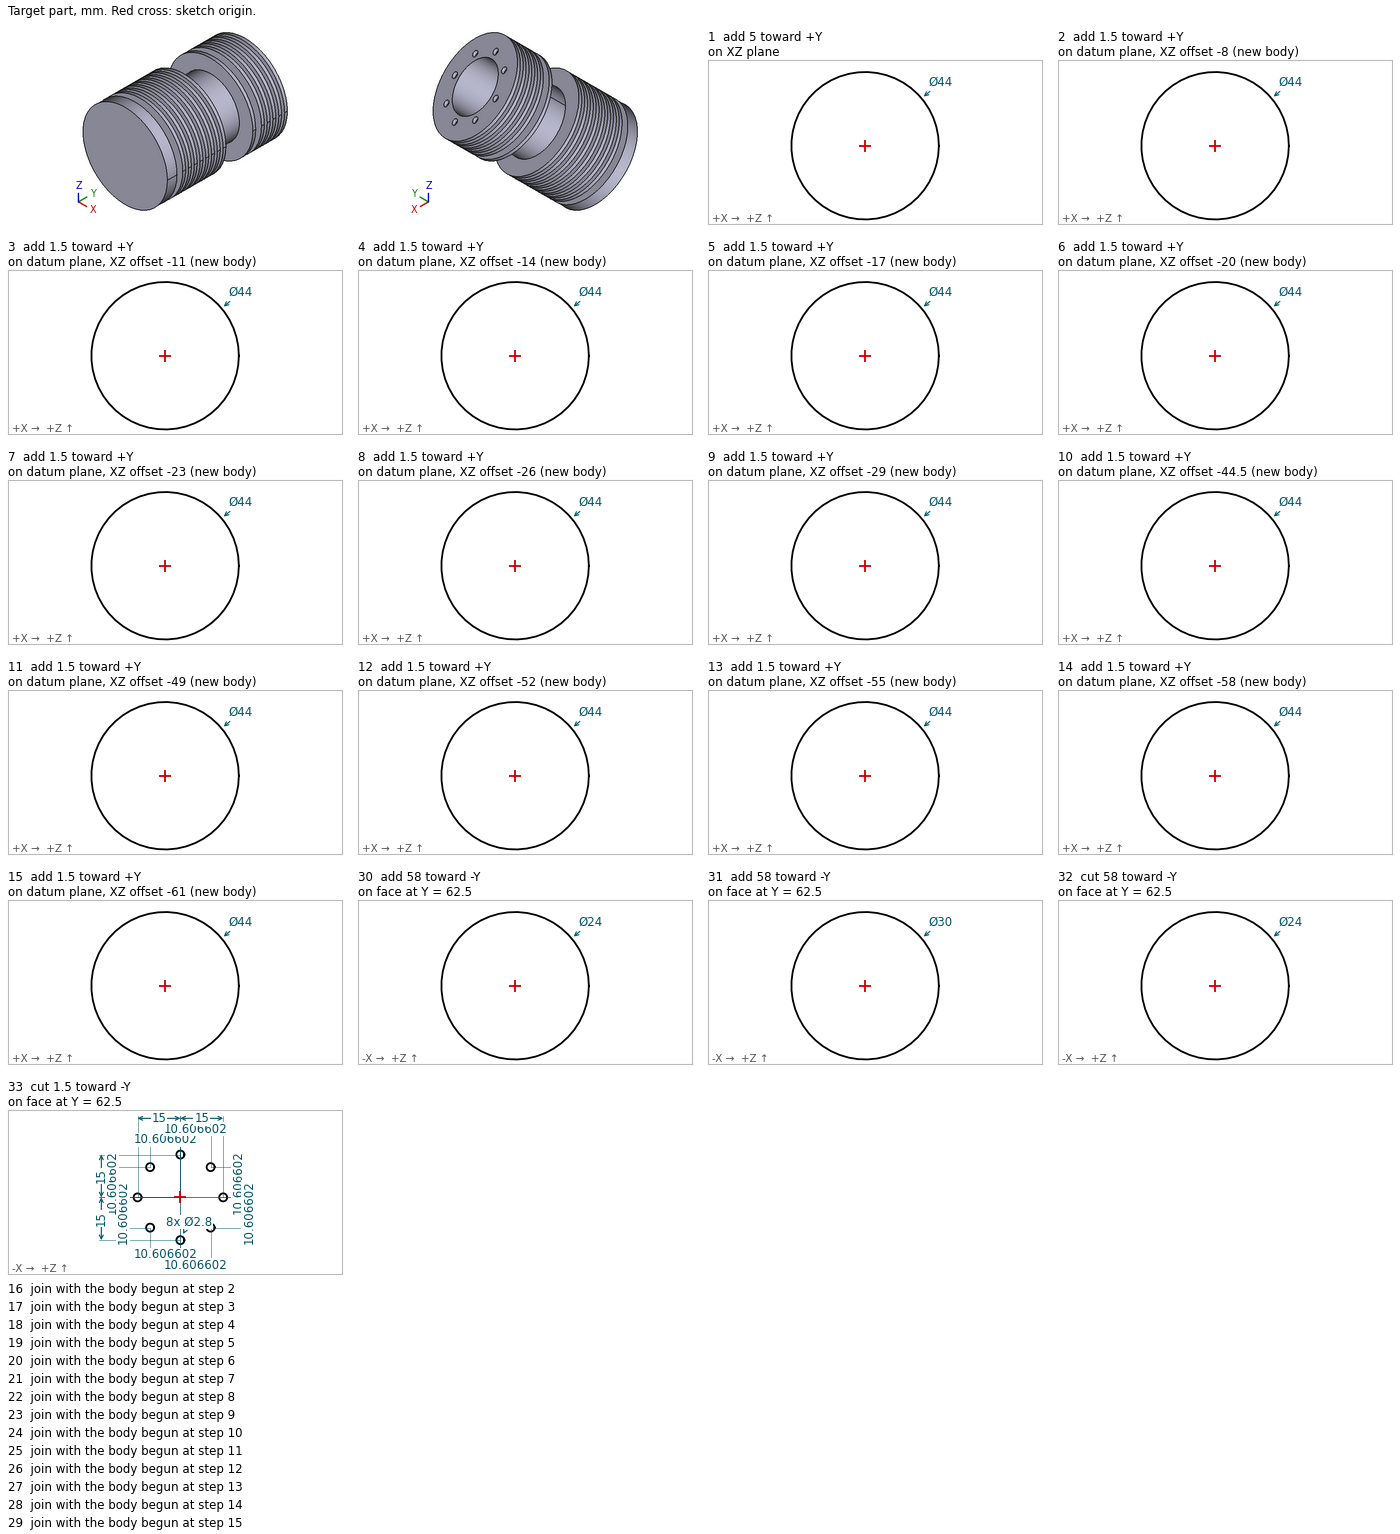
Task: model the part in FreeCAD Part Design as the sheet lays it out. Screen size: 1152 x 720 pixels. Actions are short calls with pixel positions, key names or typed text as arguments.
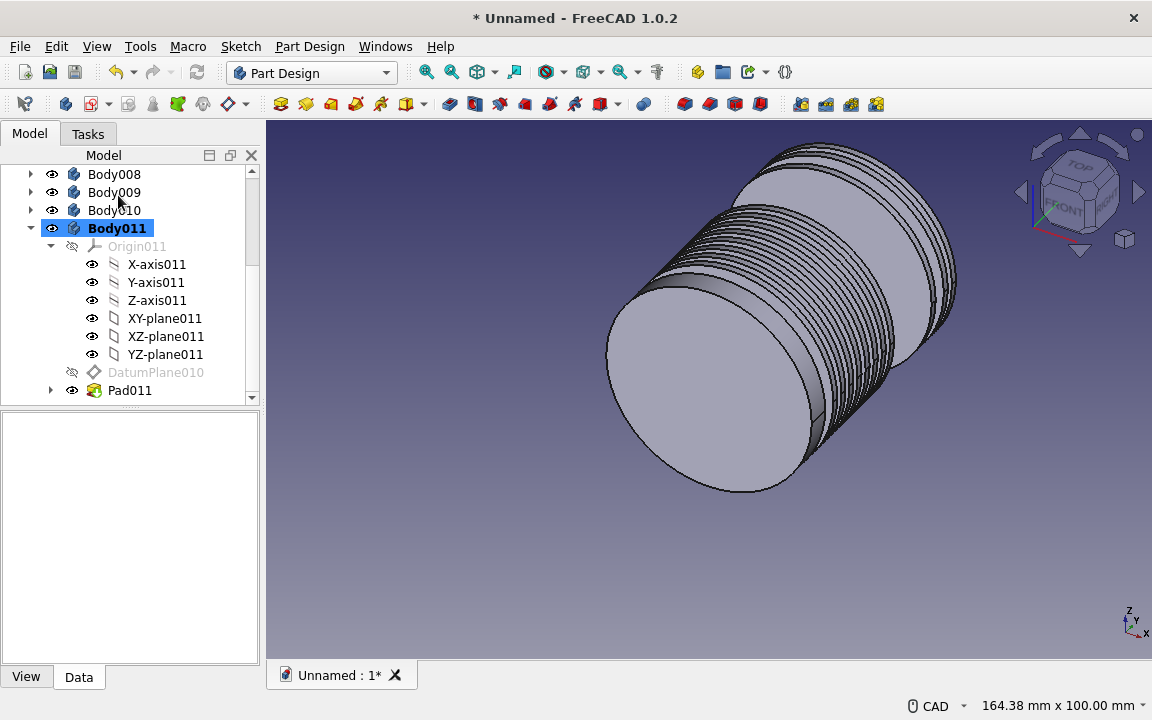
key(v)
key(f)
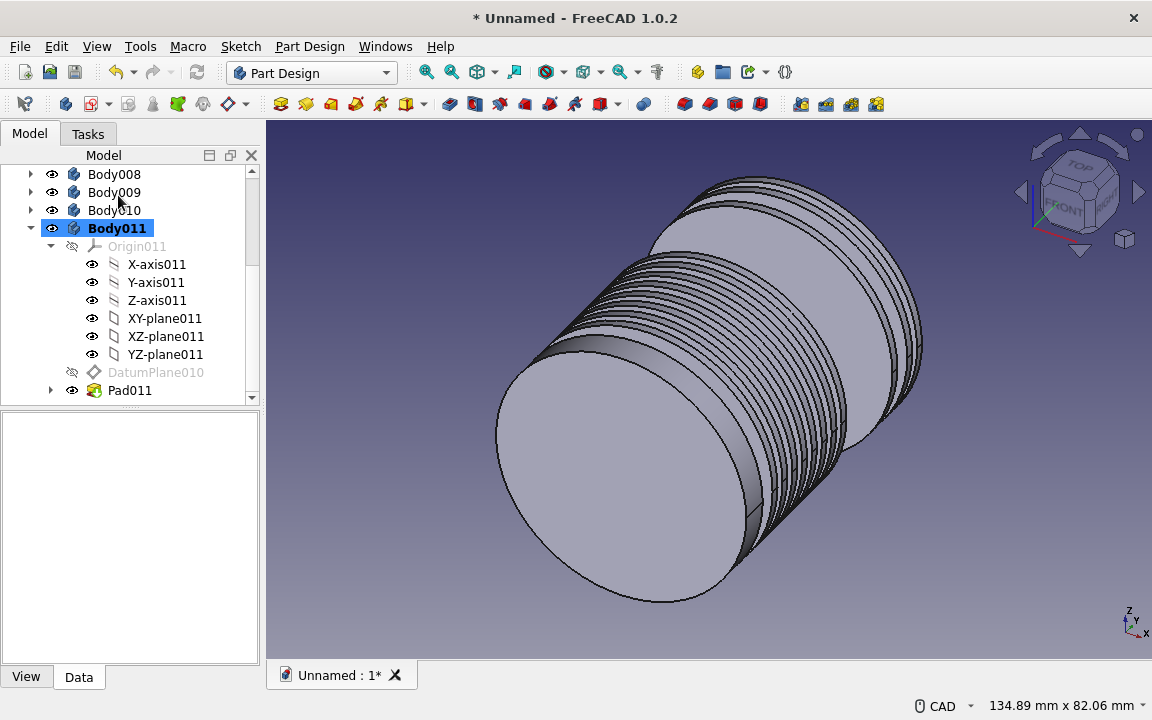
click(66, 104)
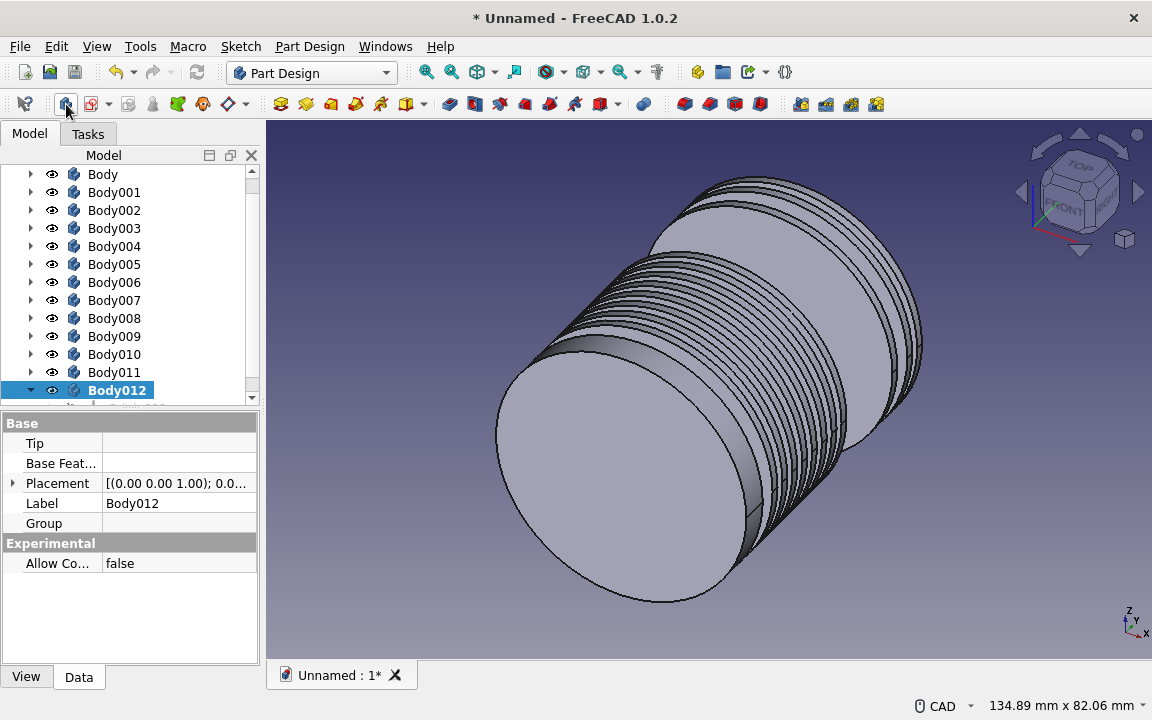
scroll(121, 278, down, 3)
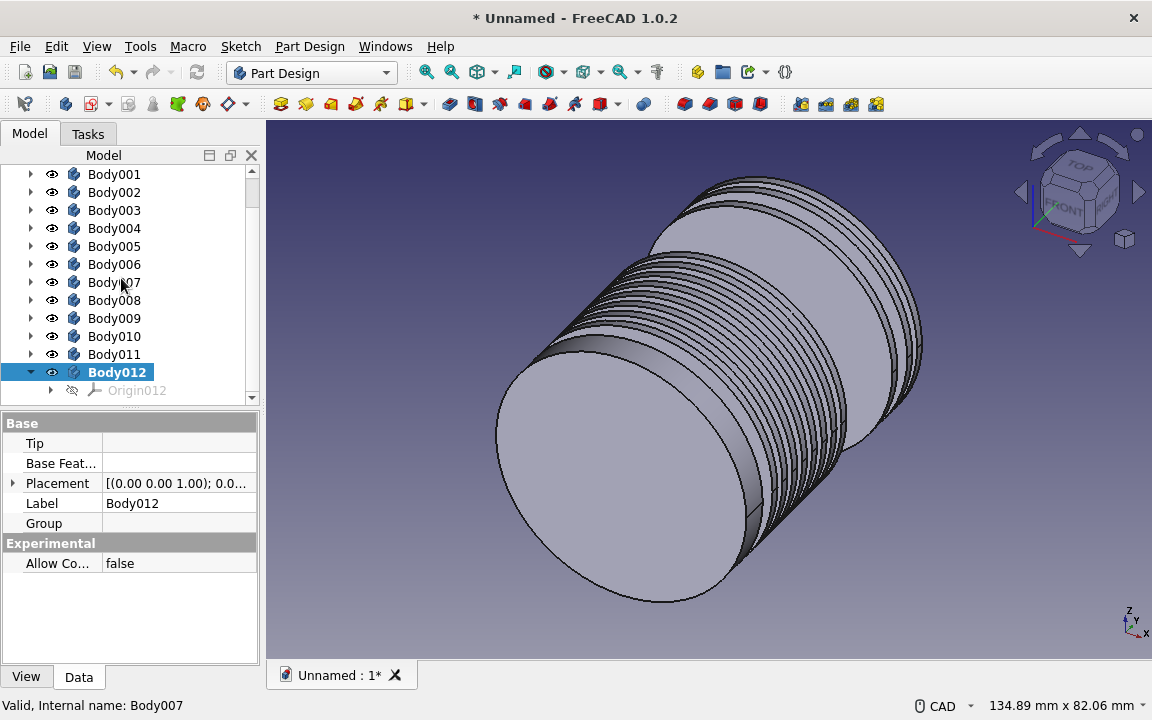
click(51, 390)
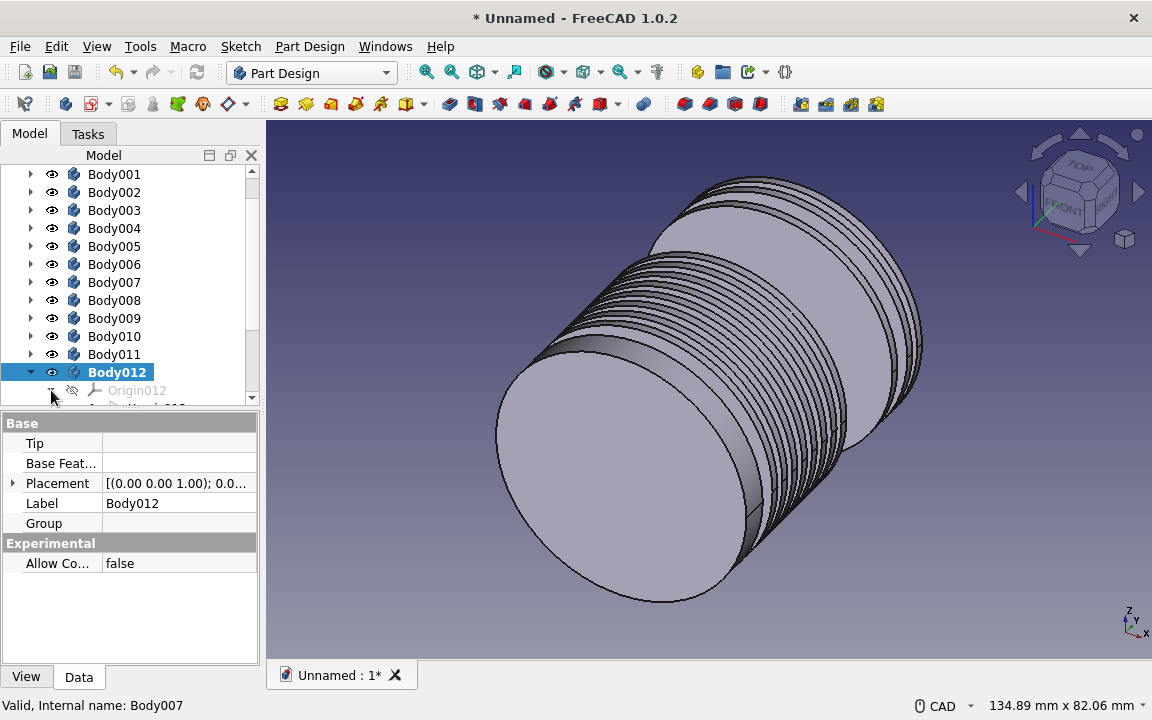
scroll(121, 278, down, 3)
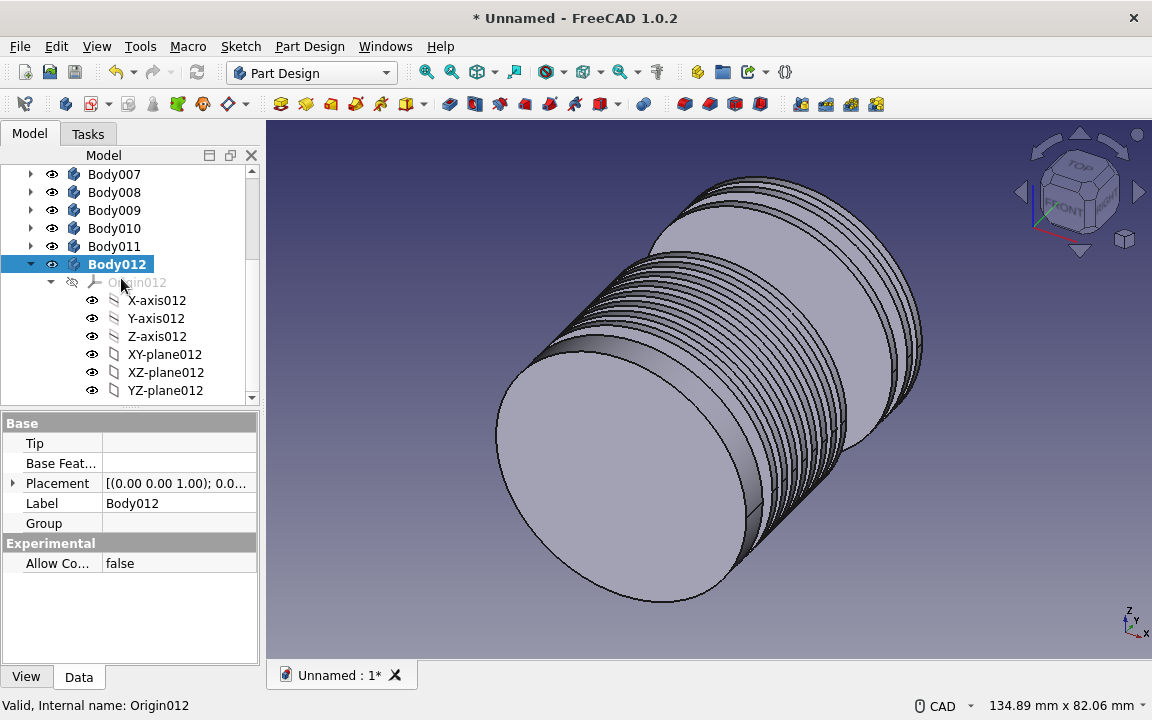
click(137, 372)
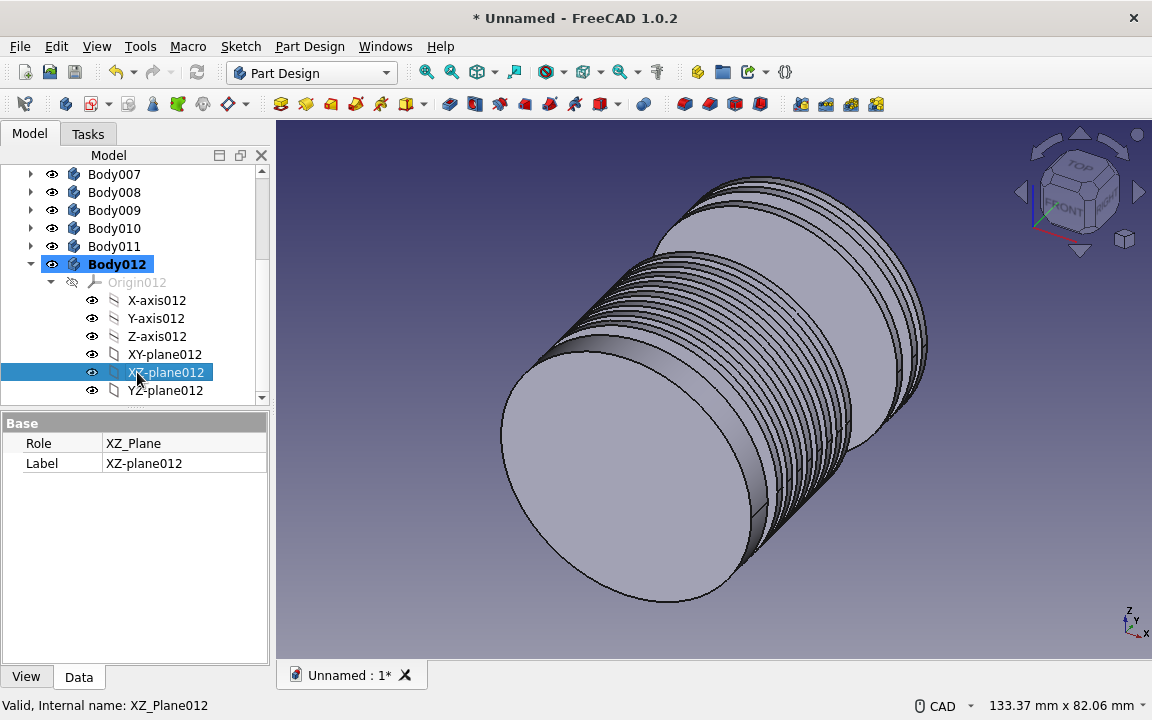
click(228, 104)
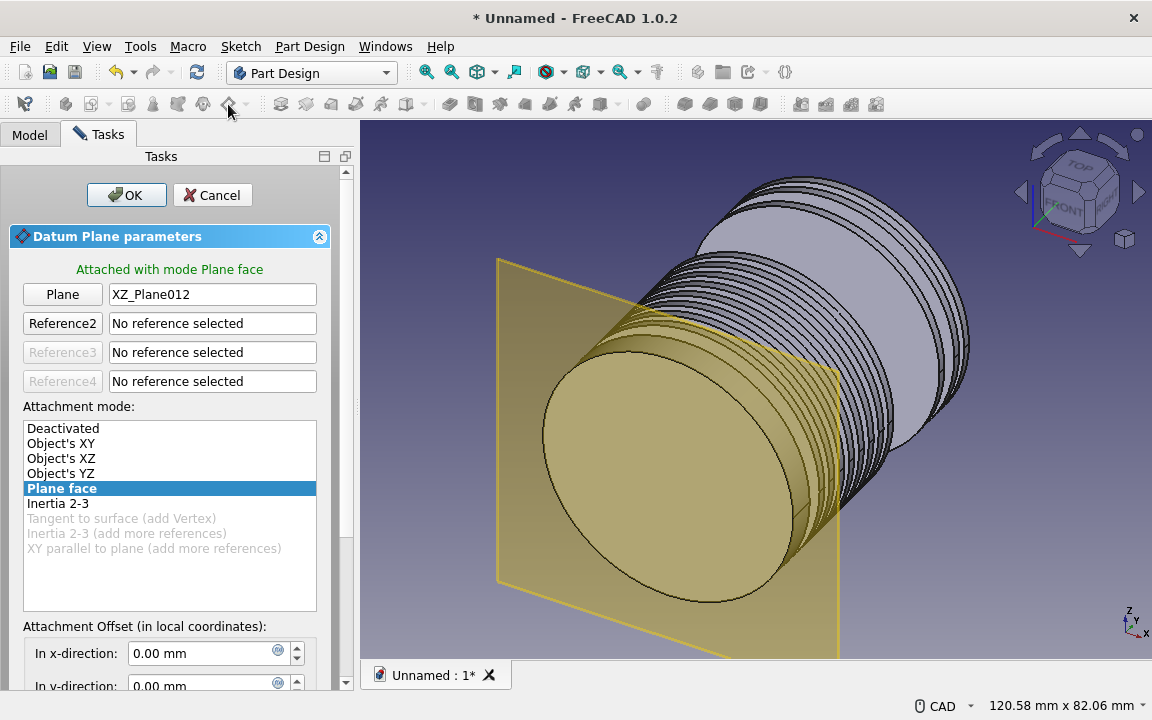
scroll(346, 428, down, 2)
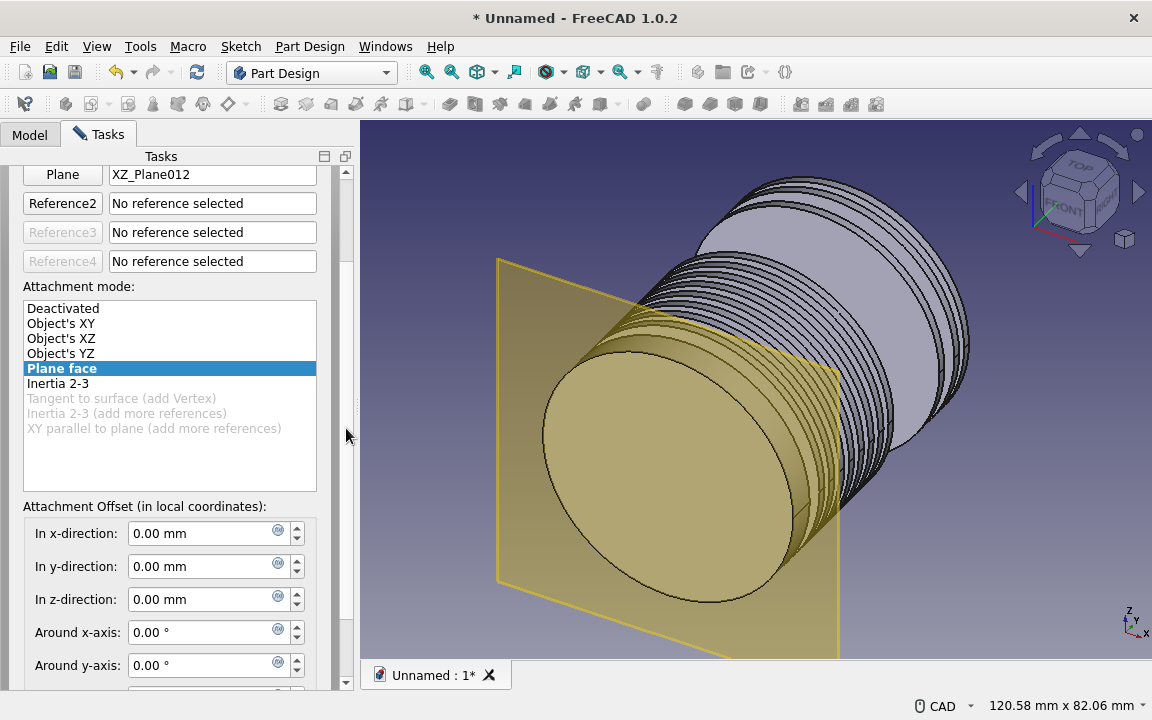
triple_click(210, 600)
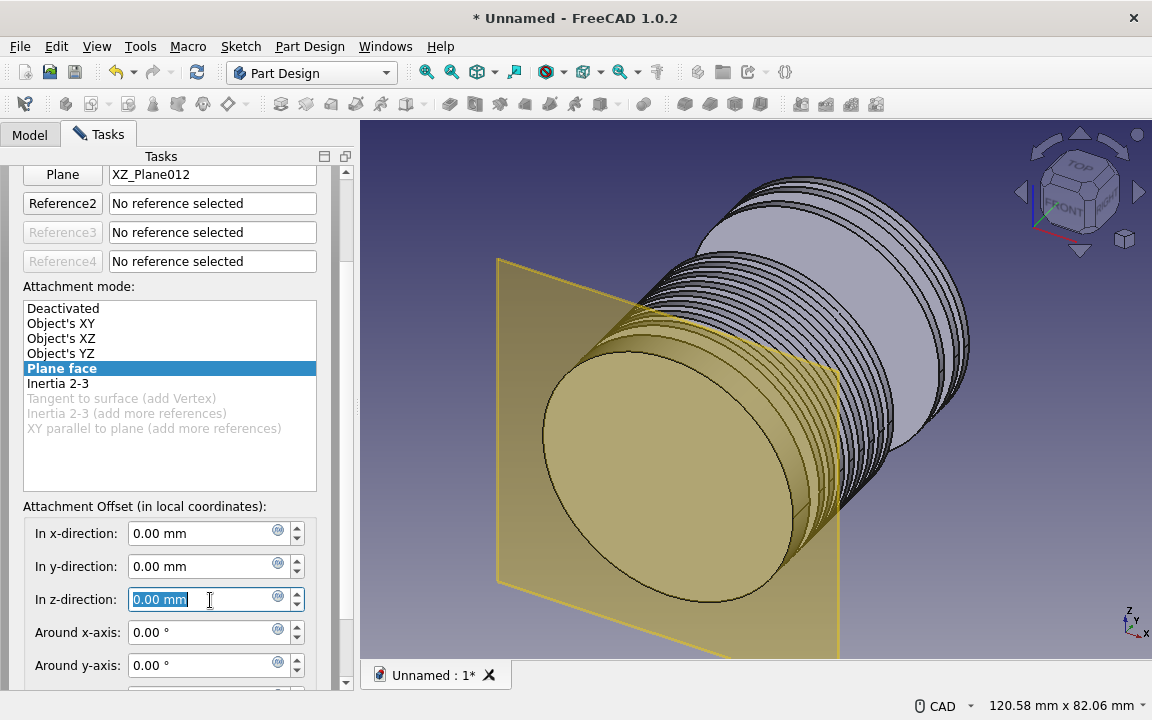
text(-55)
key(Tab)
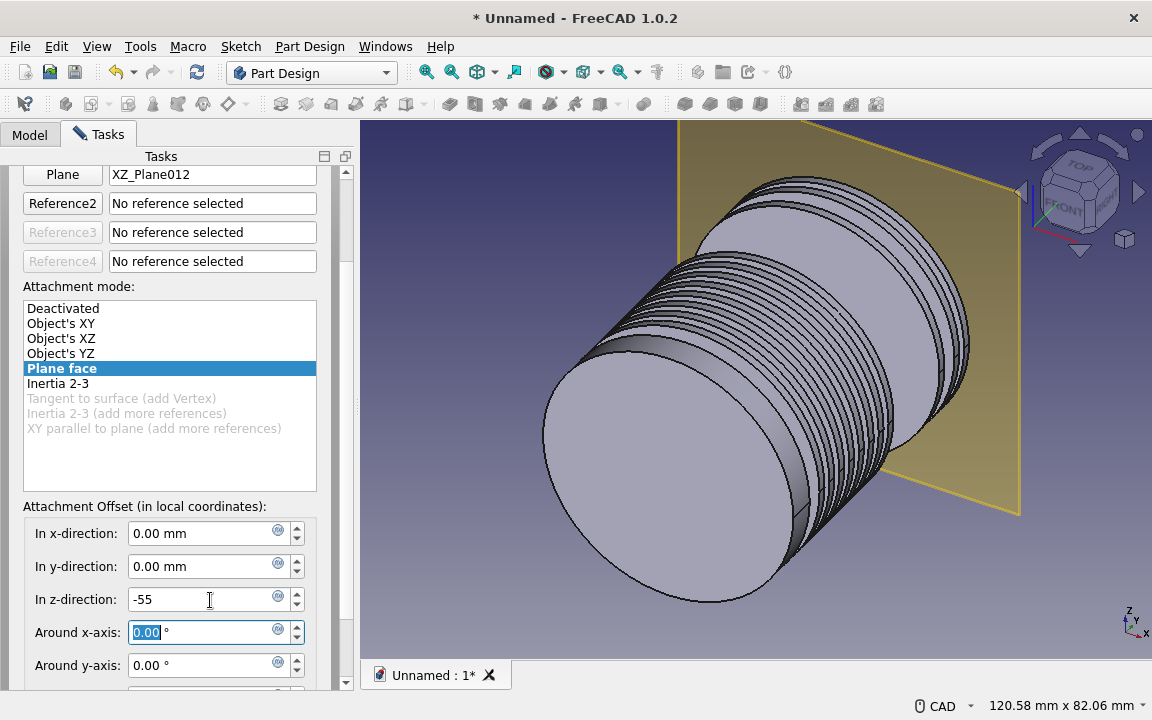
scroll(346, 428, up, 3)